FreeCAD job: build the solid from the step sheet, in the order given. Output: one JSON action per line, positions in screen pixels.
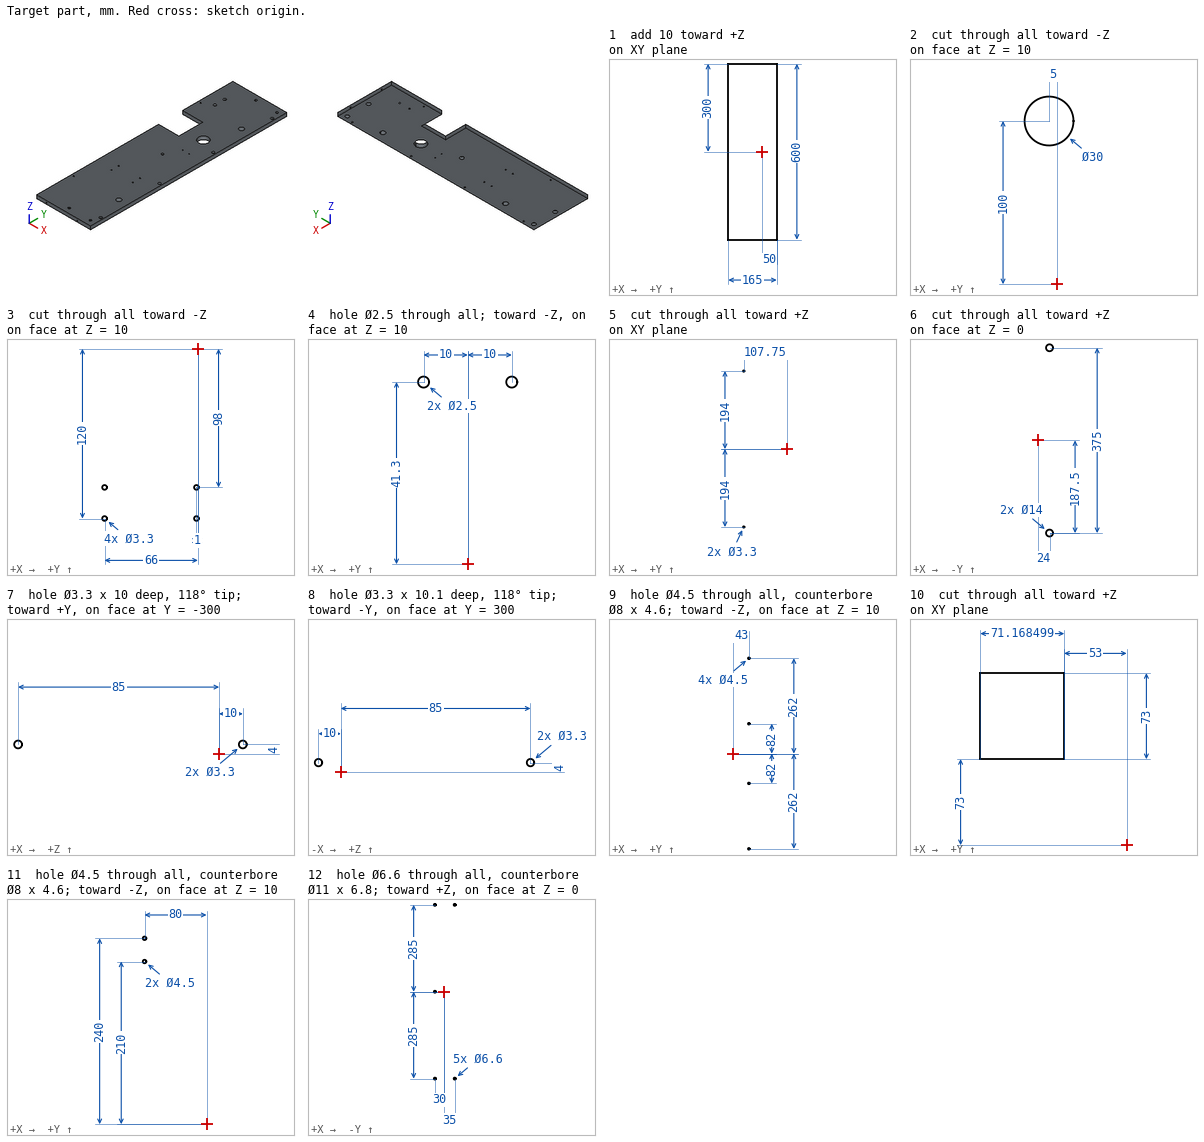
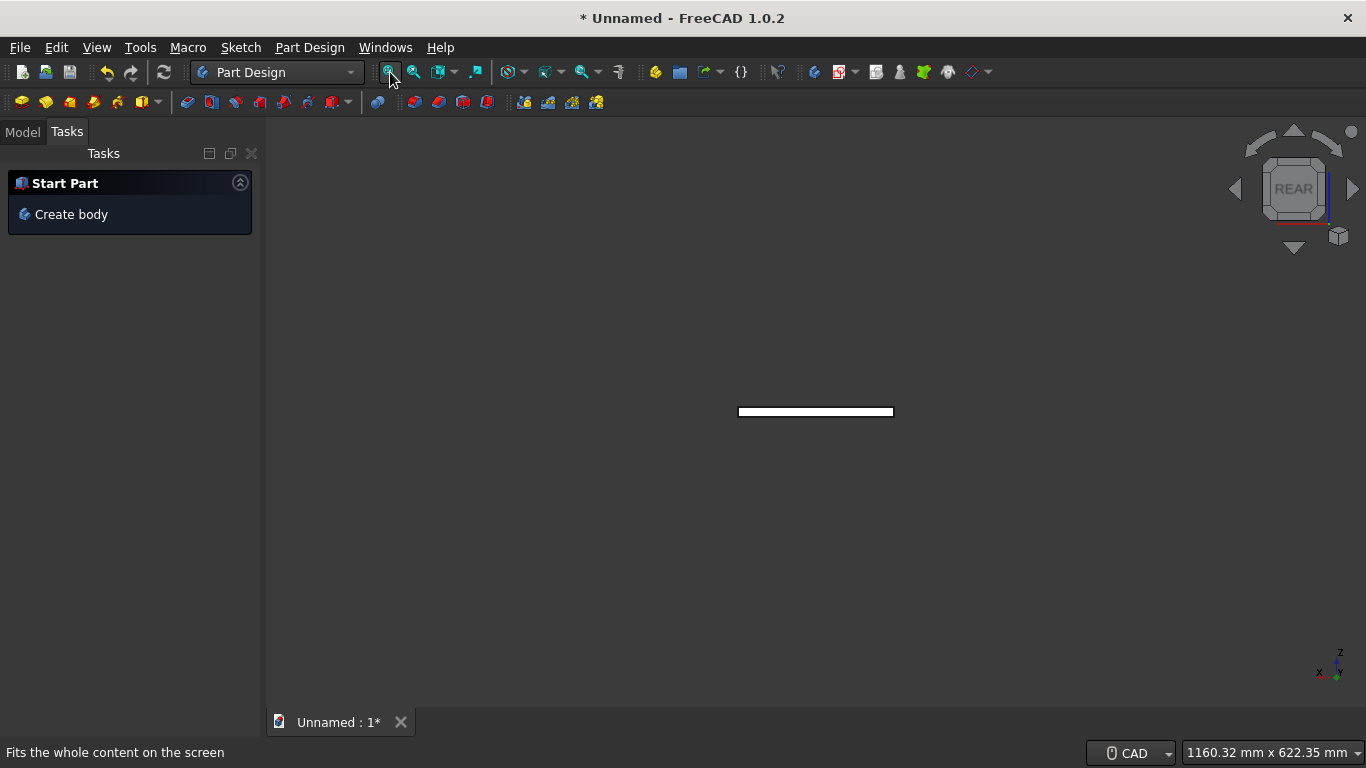
{"action": "left_click", "coordinate": [390, 72]}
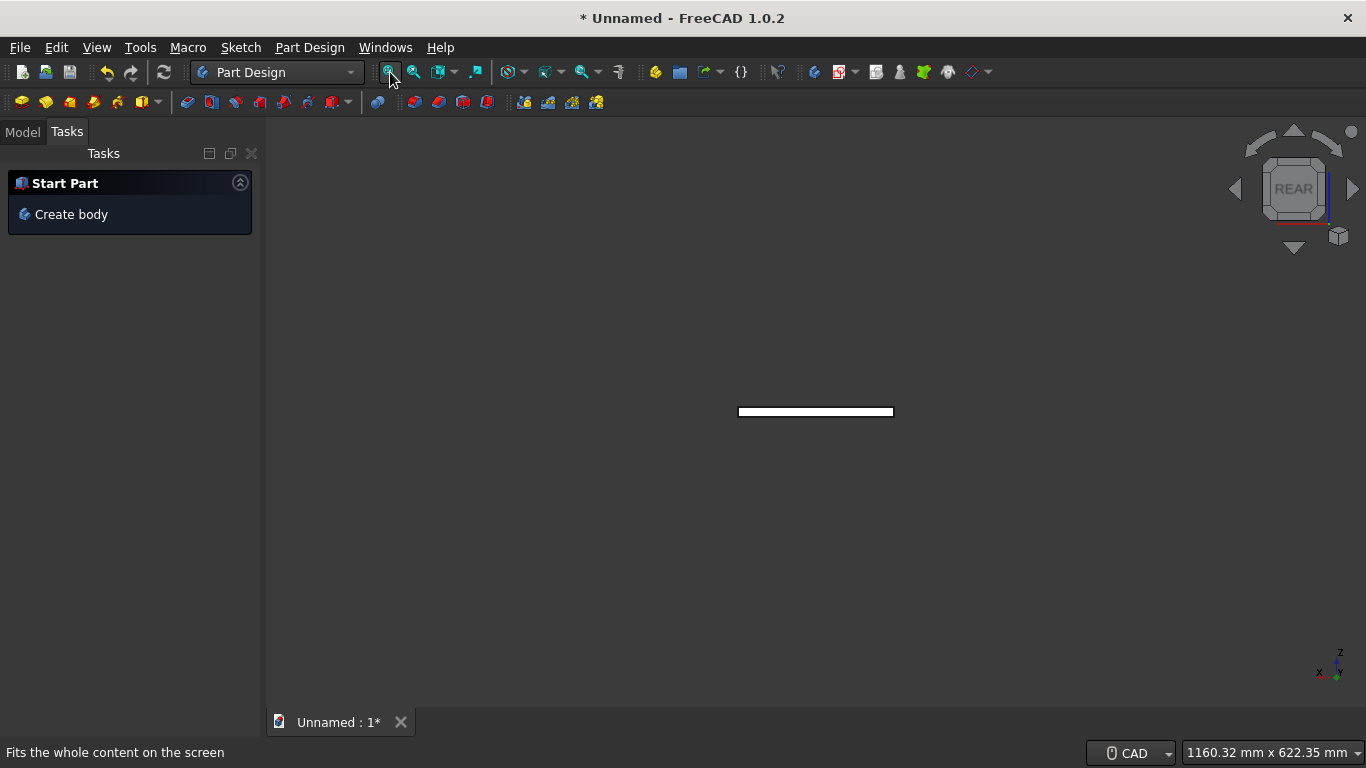
{"action": "scroll", "coordinate": [749, 411], "scroll_direction": "up", "scroll_amount": 5}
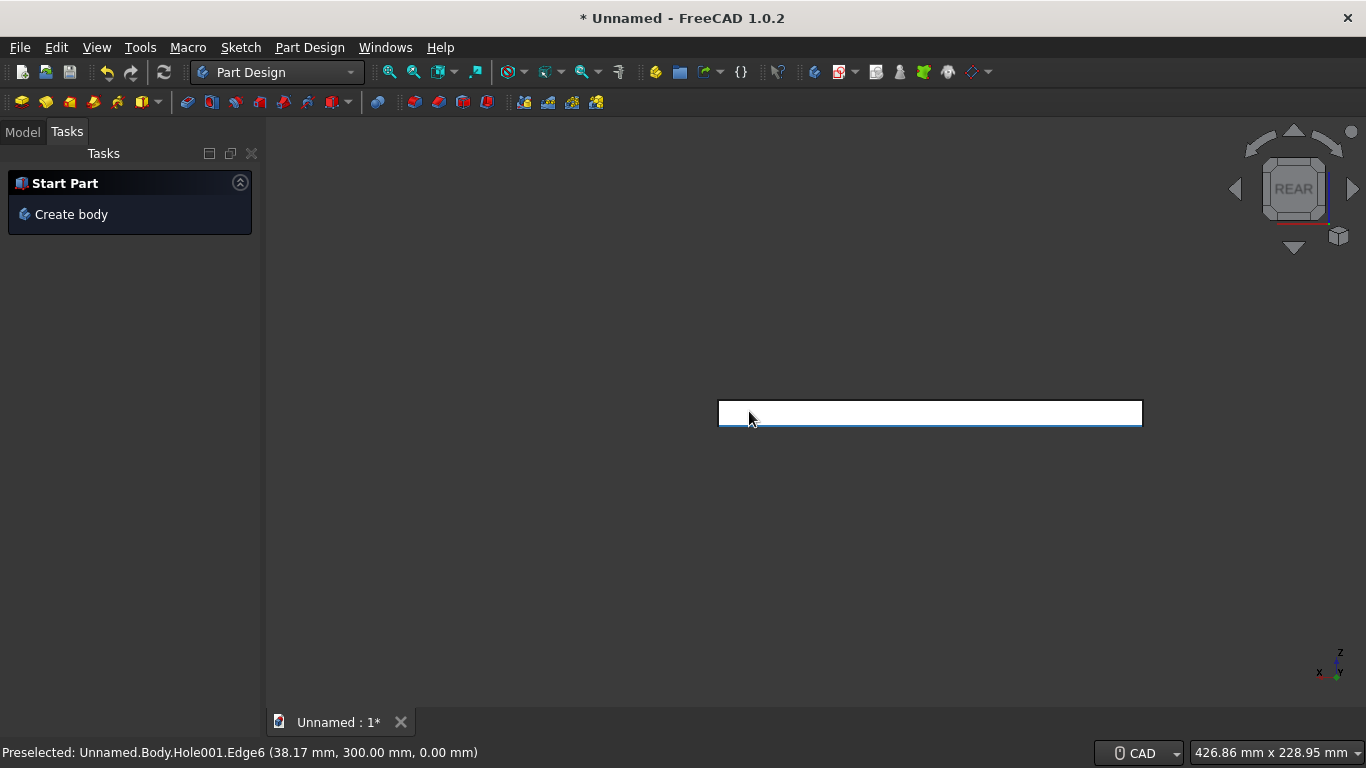
{"action": "left_click", "coordinate": [748, 412]}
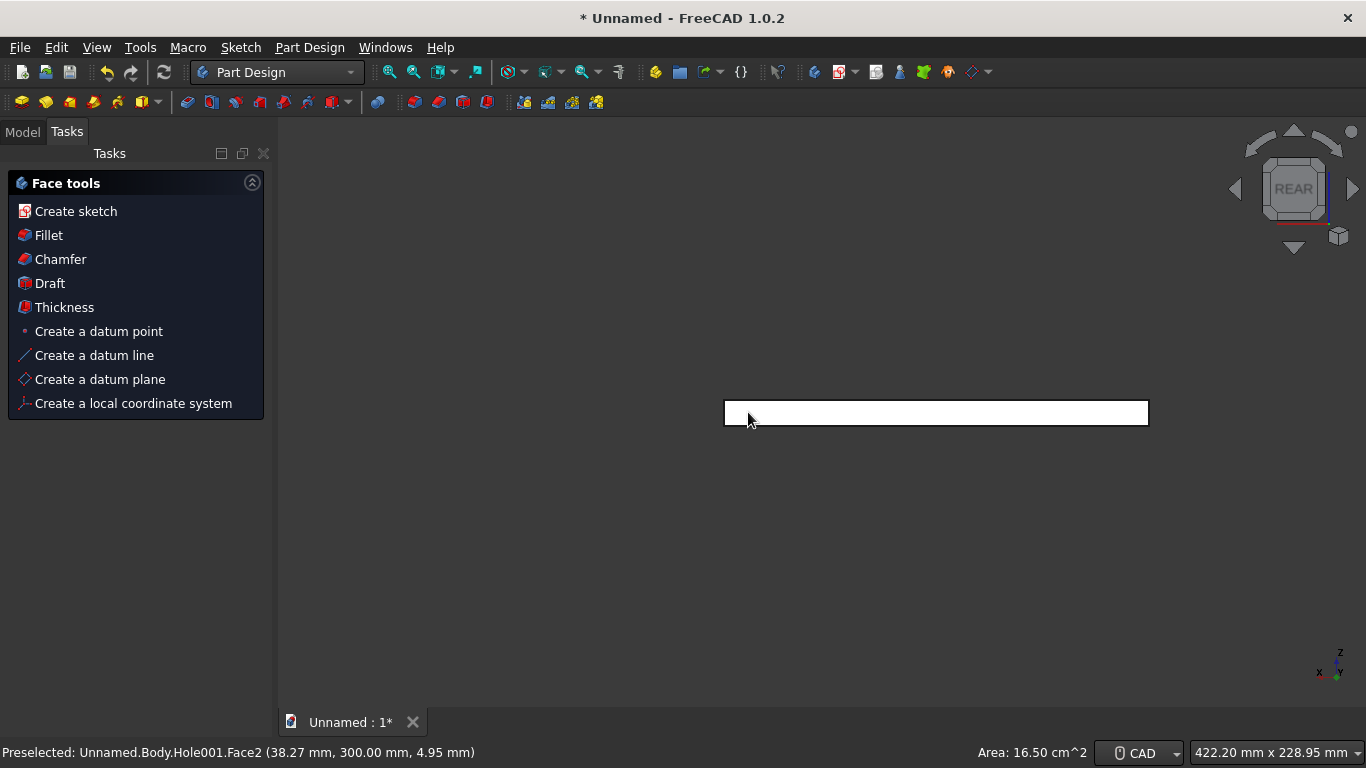
{"action": "left_click", "coordinate": [840, 72]}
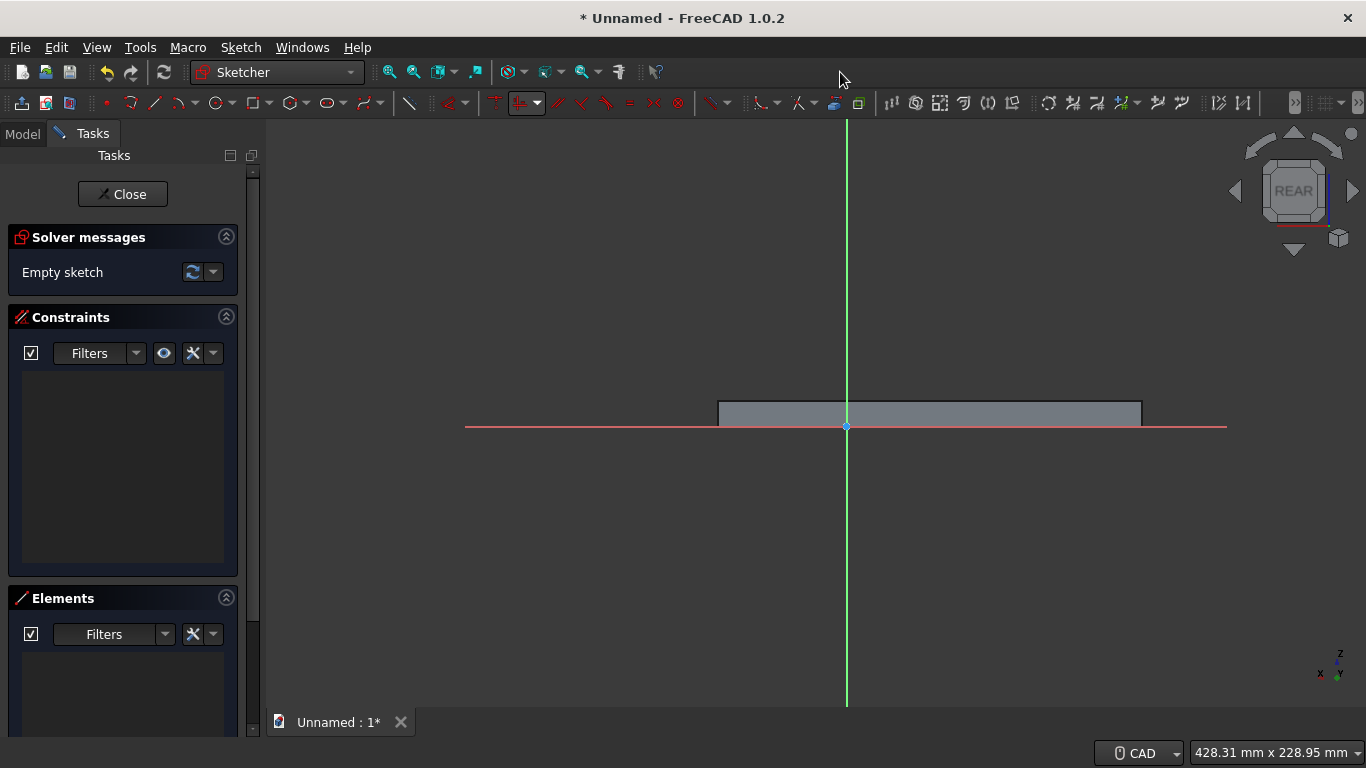
{"action": "scroll", "coordinate": [1056, 423], "scroll_direction": "up", "scroll_amount": 5}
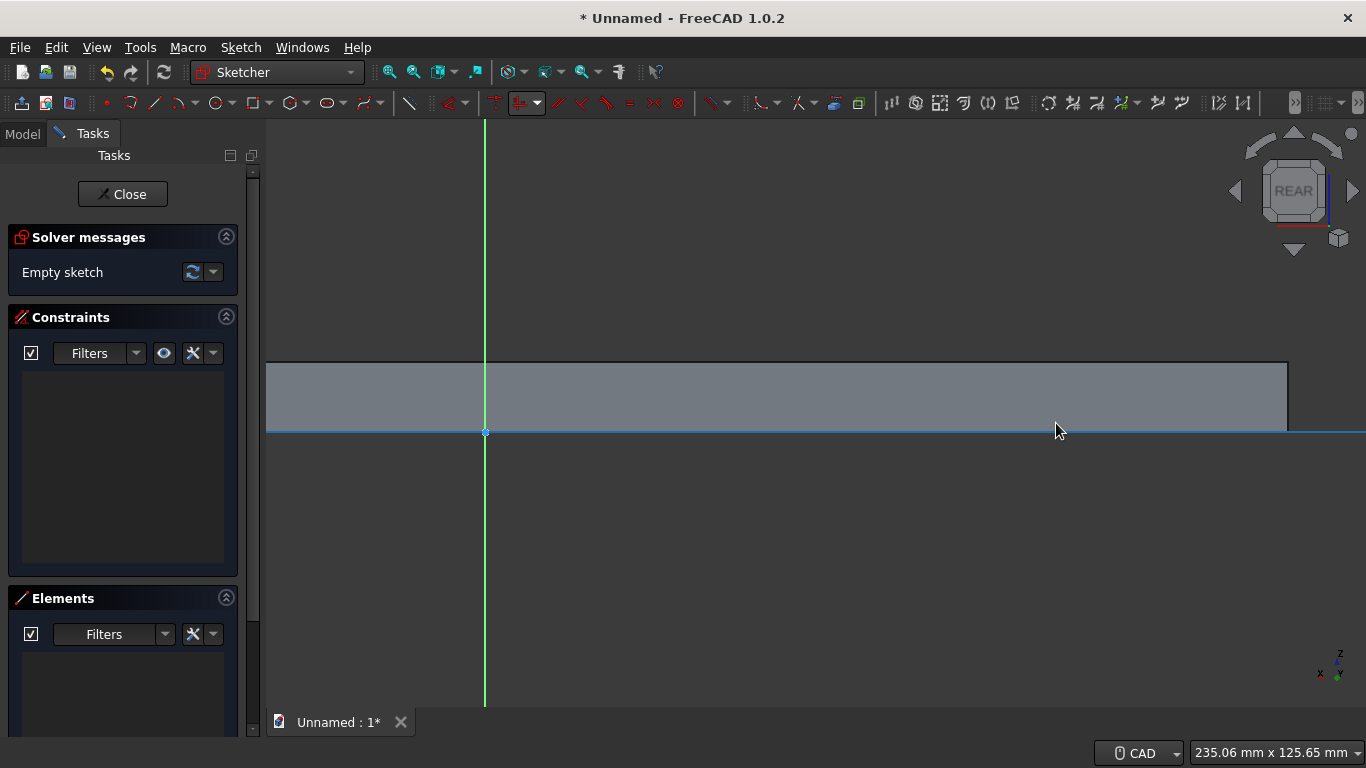
{"action": "left_click", "coordinate": [216, 104]}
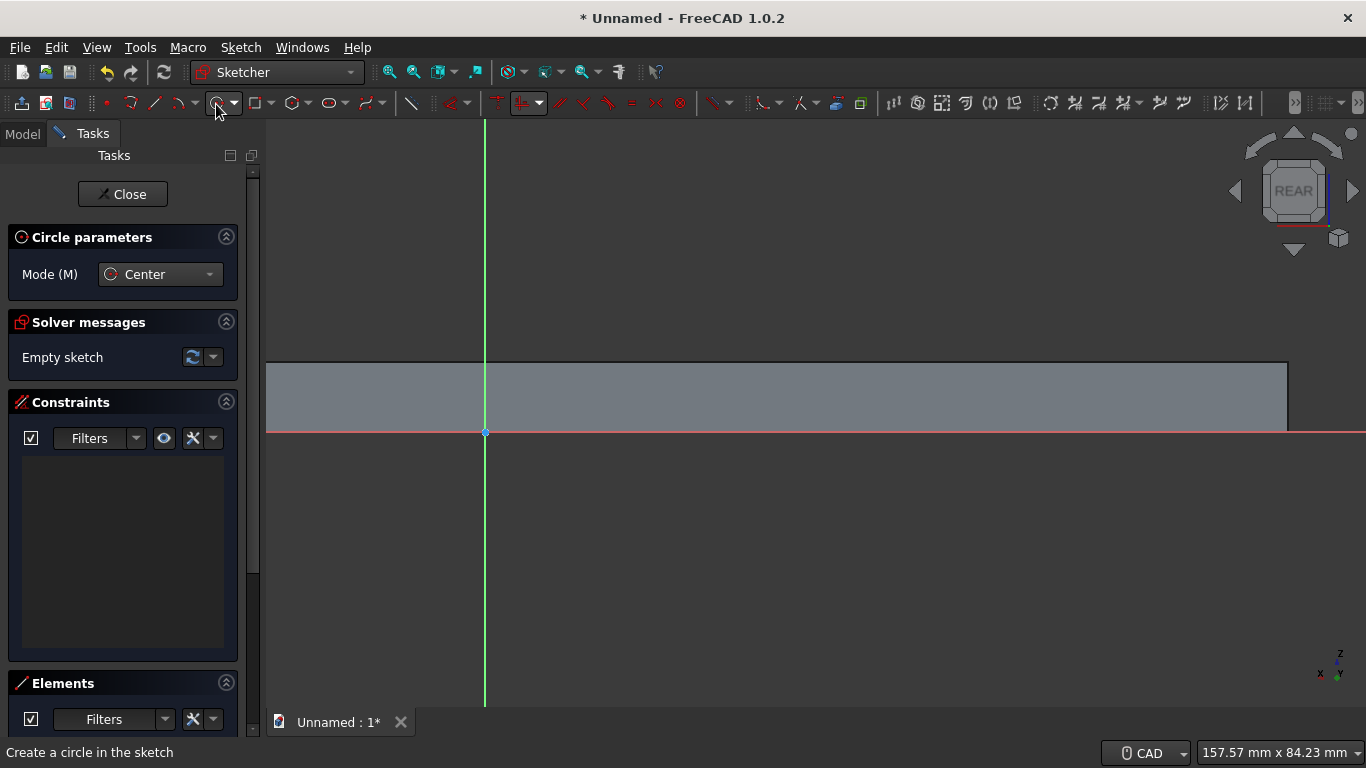
{"action": "scroll", "coordinate": [1079, 404], "scroll_direction": "up", "scroll_amount": 4}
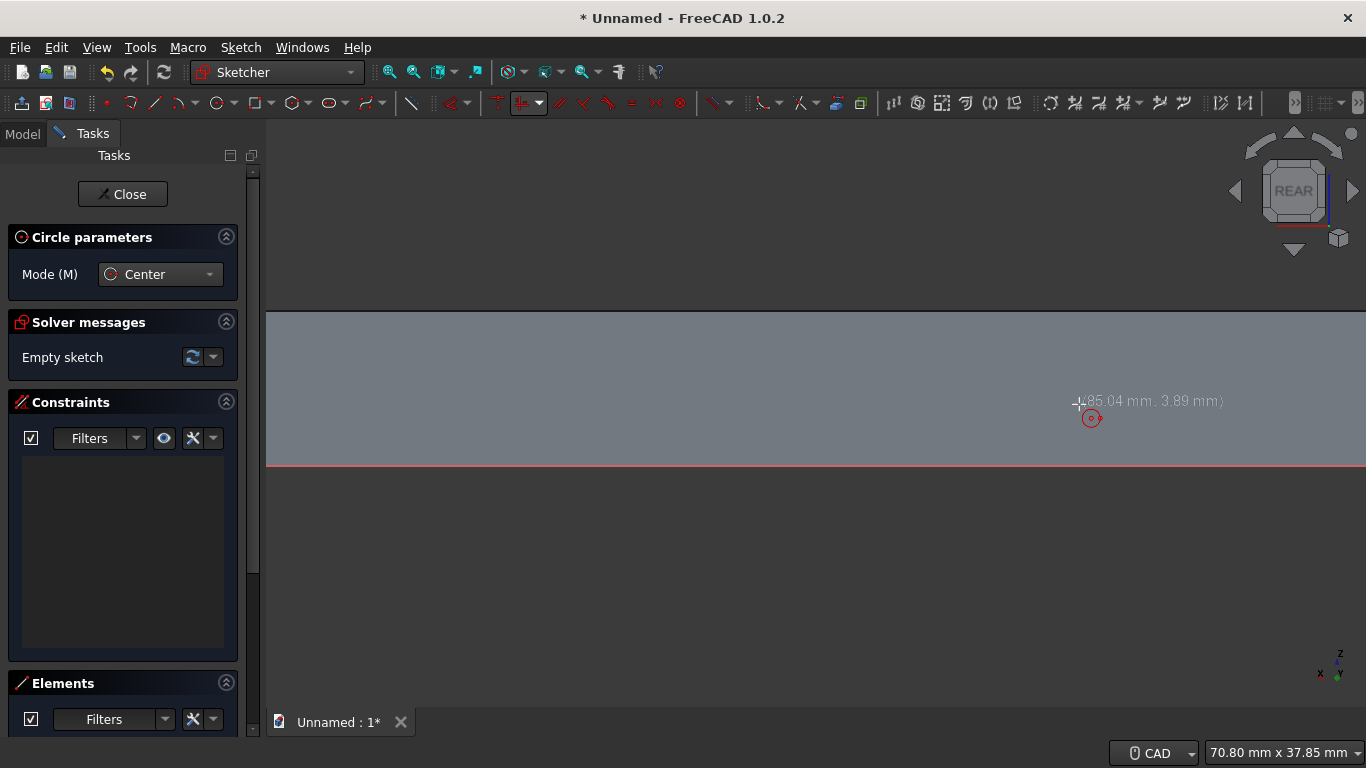
{"action": "left_click", "coordinate": [1077, 404]}
{"action": "mouse_move", "coordinate": [1096, 386]}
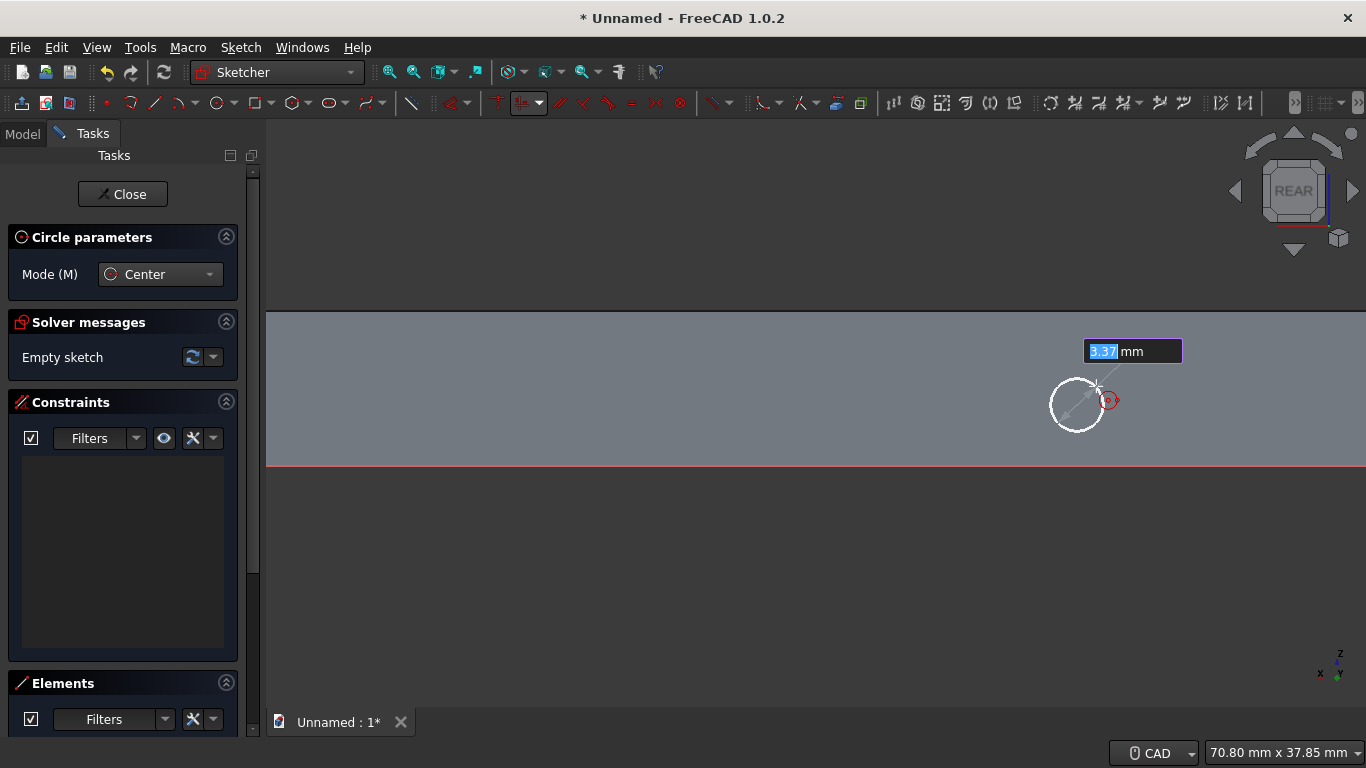
{"action": "type", "text": "3.3"}
{"action": "key", "text": "Return"}